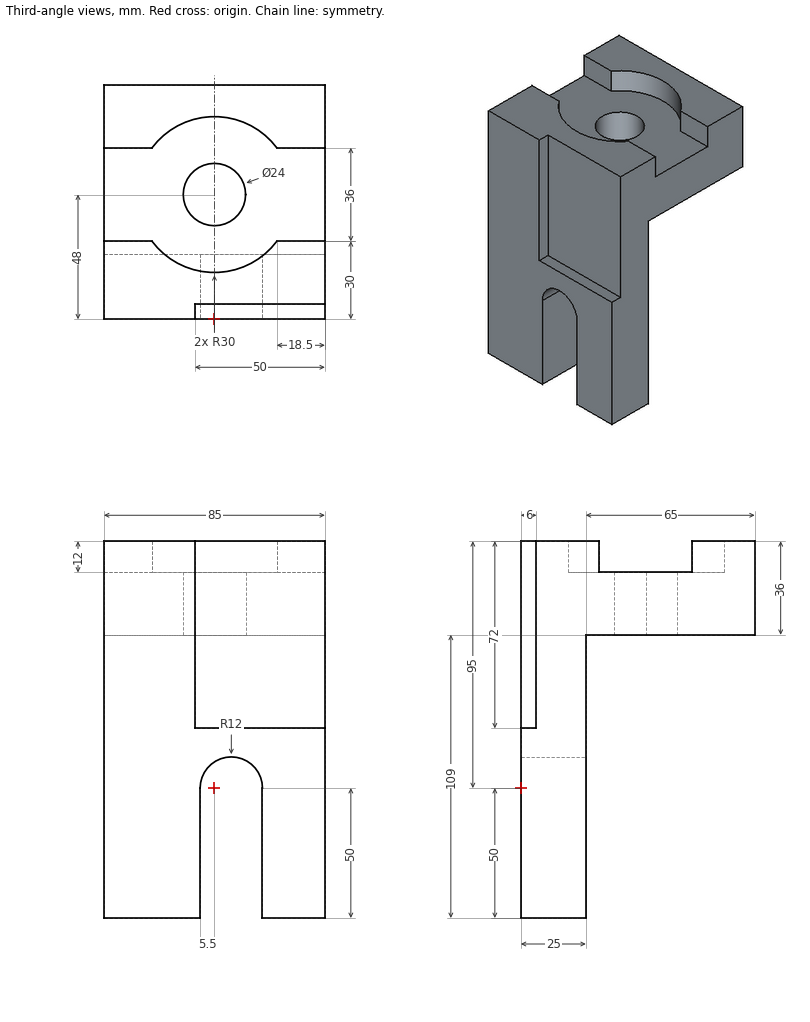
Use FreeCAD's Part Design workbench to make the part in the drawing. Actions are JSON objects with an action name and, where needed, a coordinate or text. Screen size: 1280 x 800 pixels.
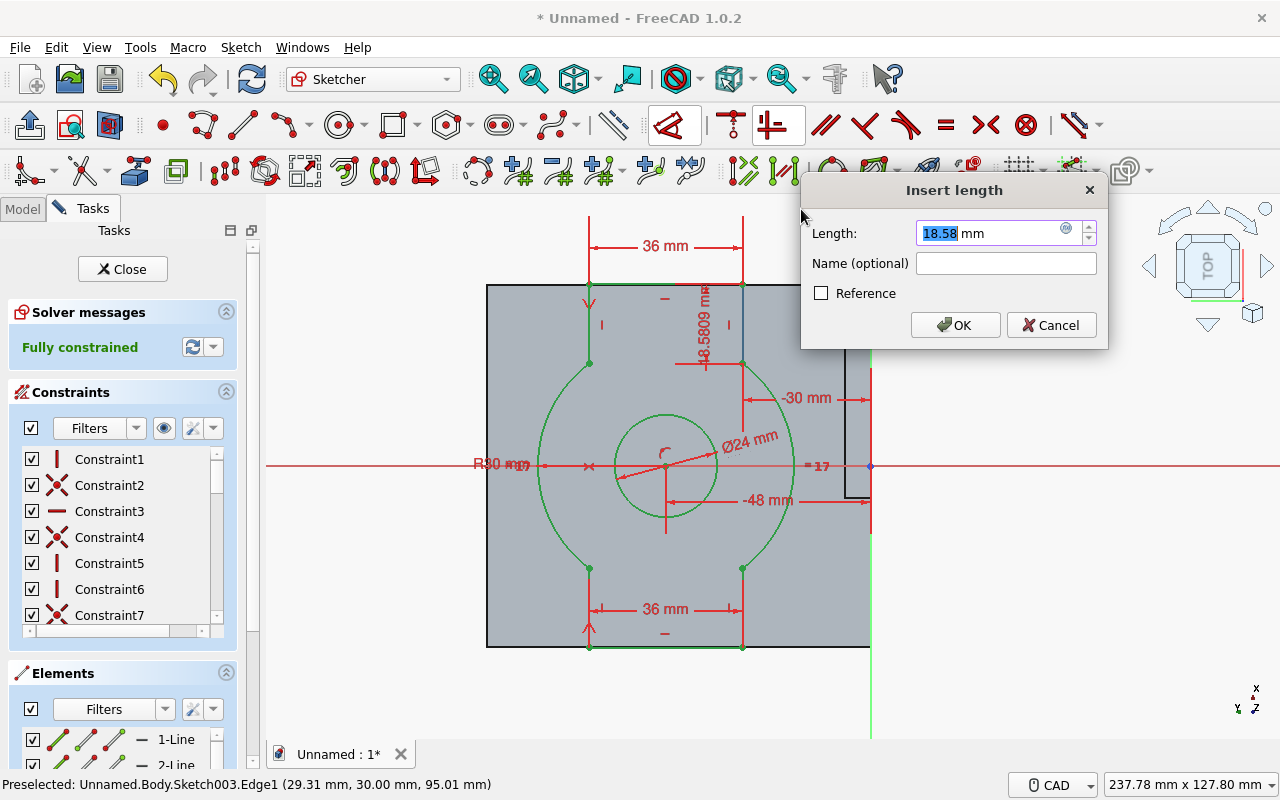
{"action": "type", "text": "18.5"}
{"action": "key", "text": "Return"}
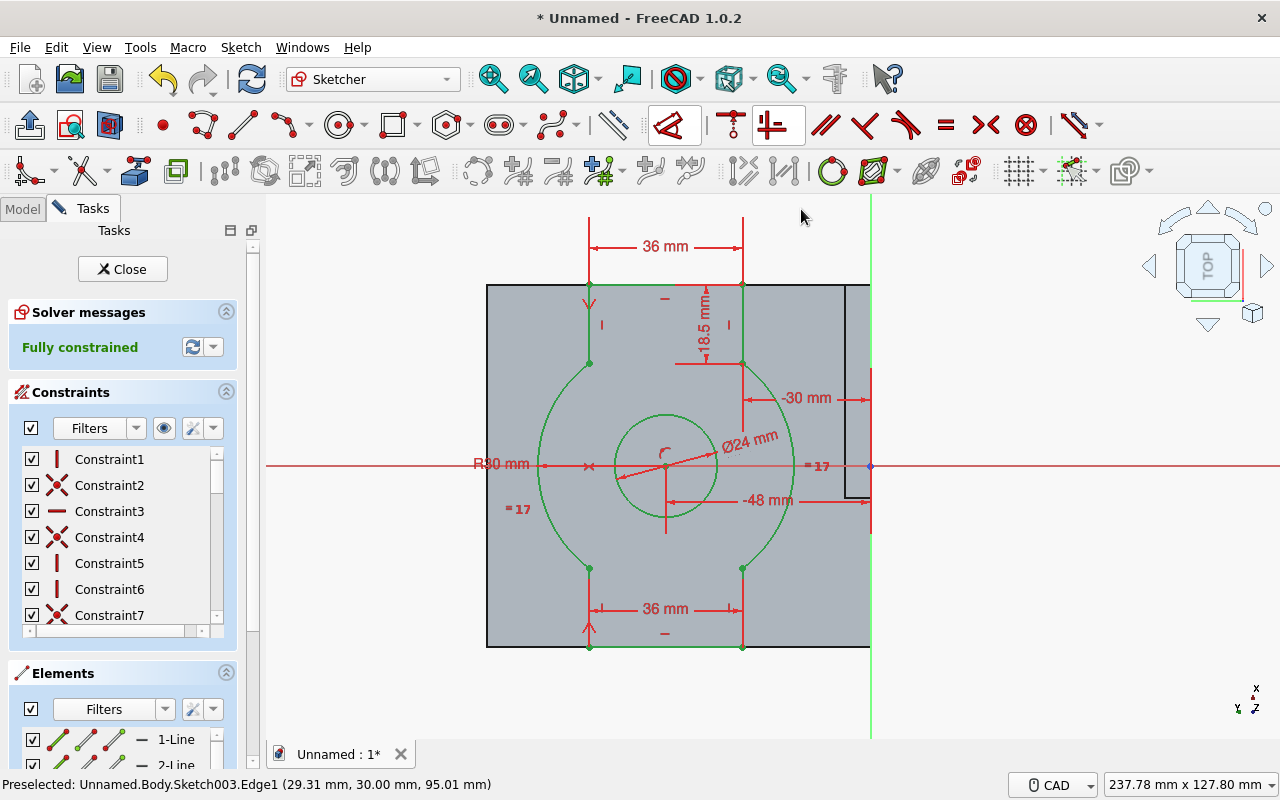
{"action": "left_click", "coordinate": [123, 269]}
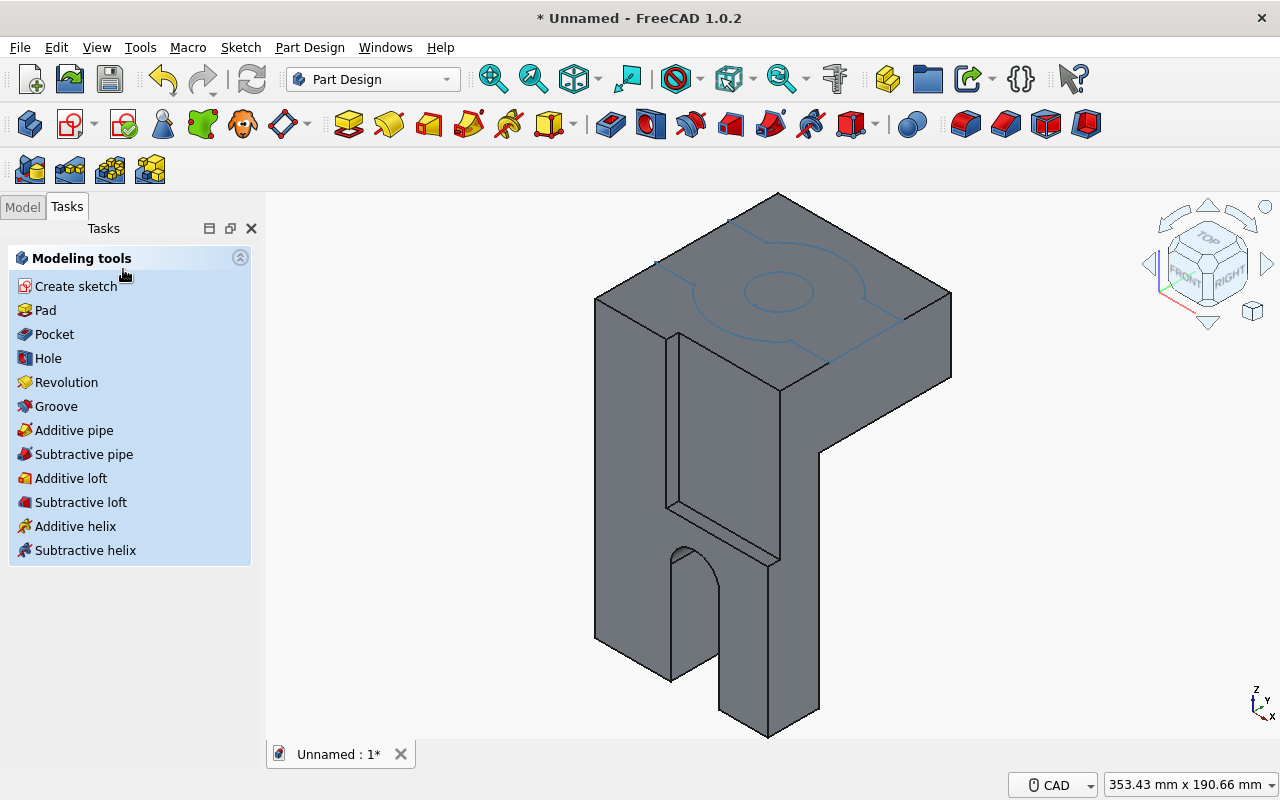
{"action": "left_click", "coordinate": [612, 124]}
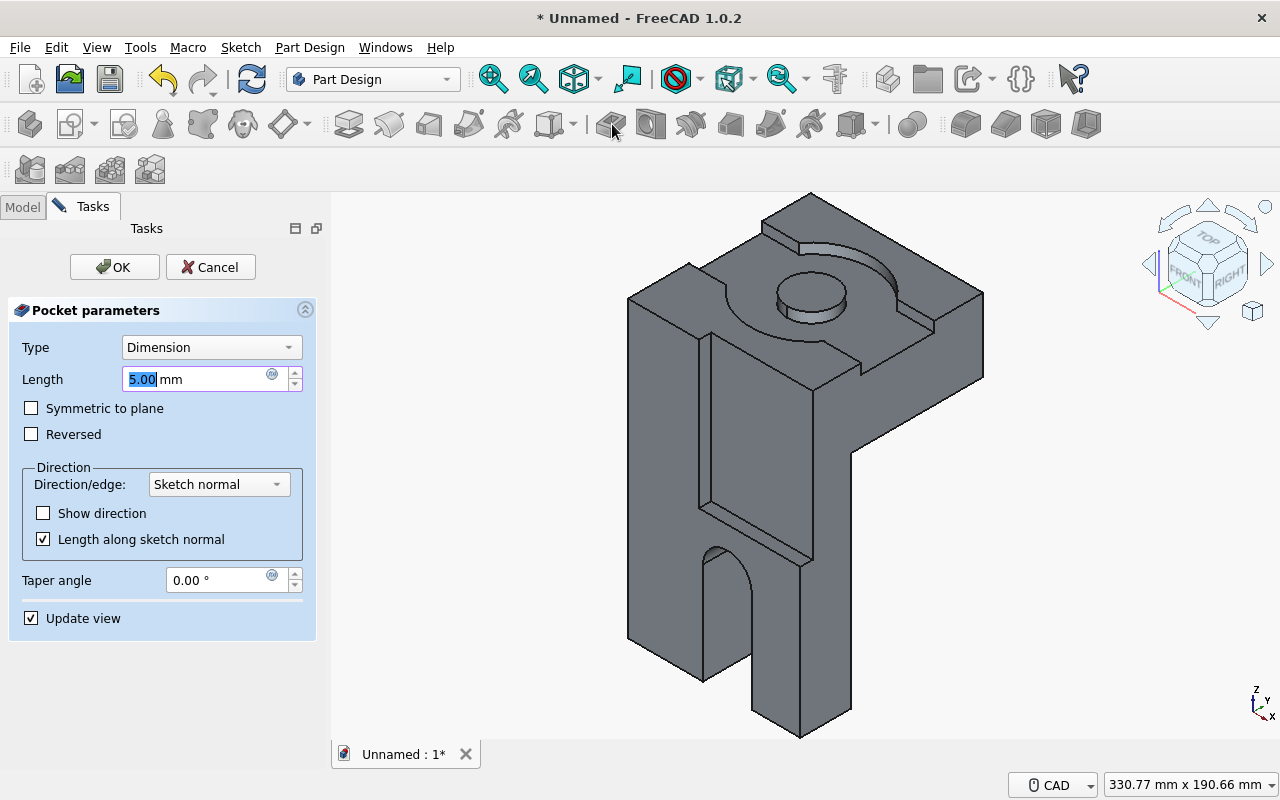
{"action": "type", "text": "12"}
{"action": "key", "text": "Tab"}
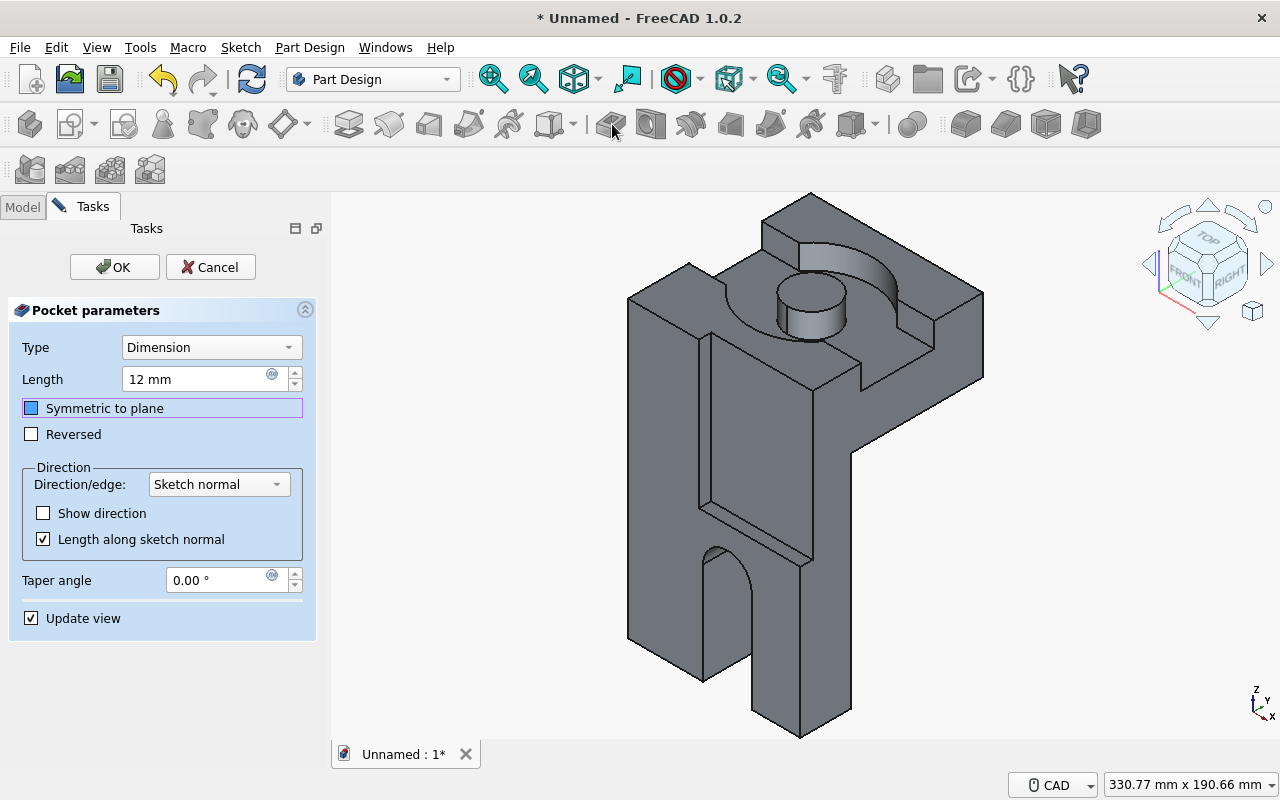
{"action": "left_click", "coordinate": [115, 267]}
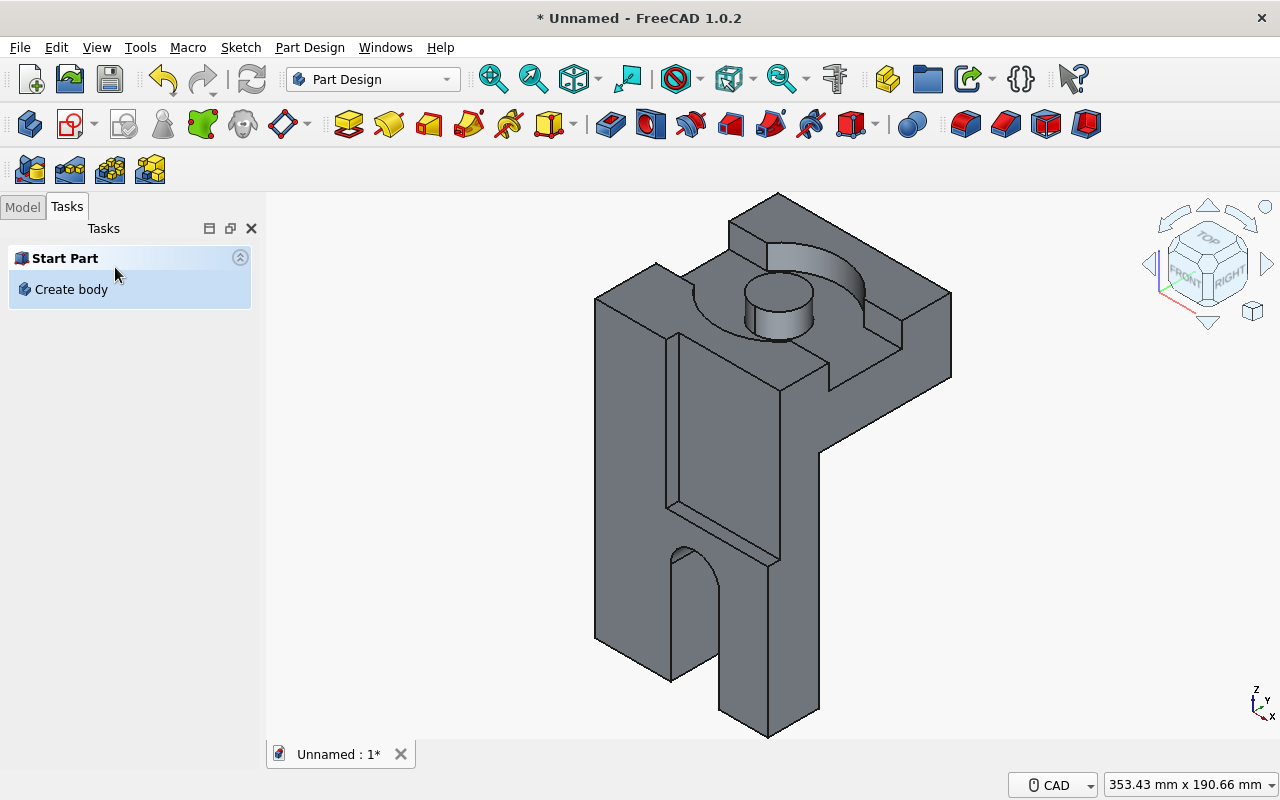
{"action": "left_click", "coordinate": [663, 301]}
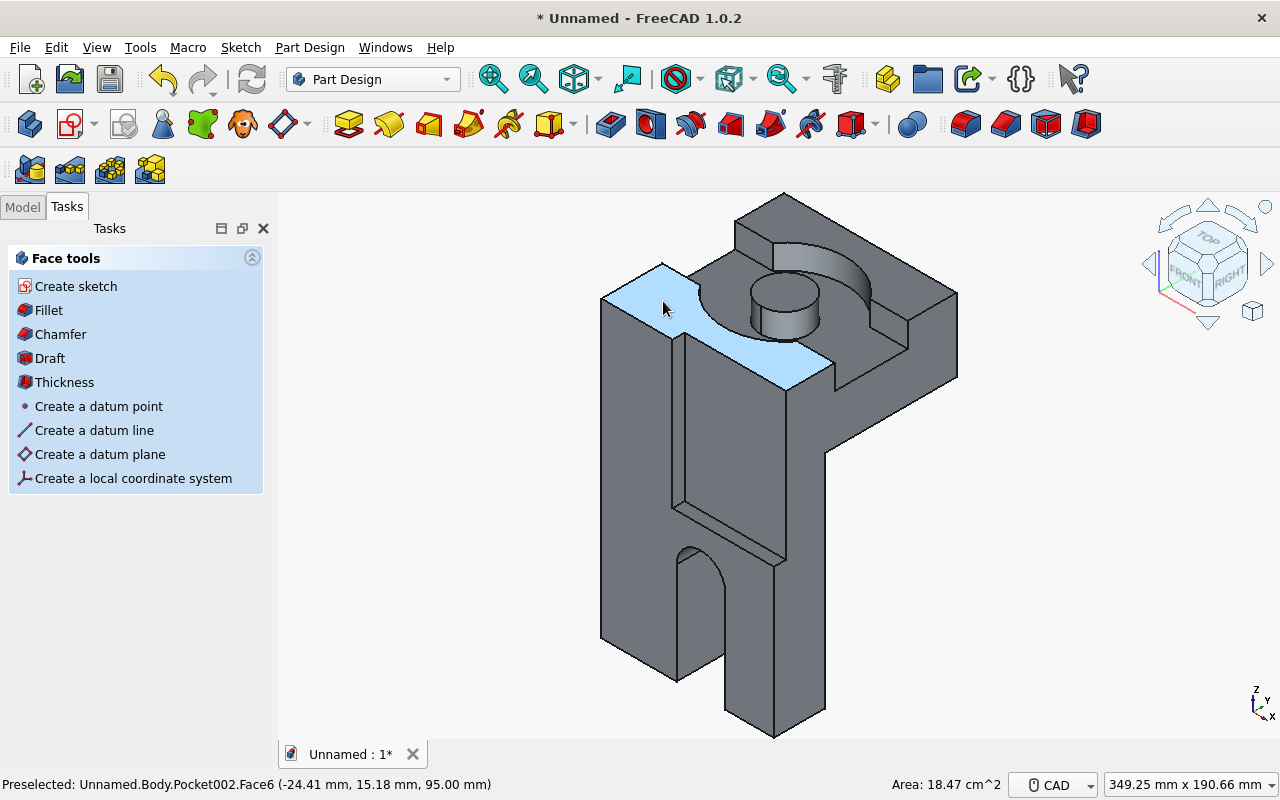
{"action": "left_click", "coordinate": [70, 124]}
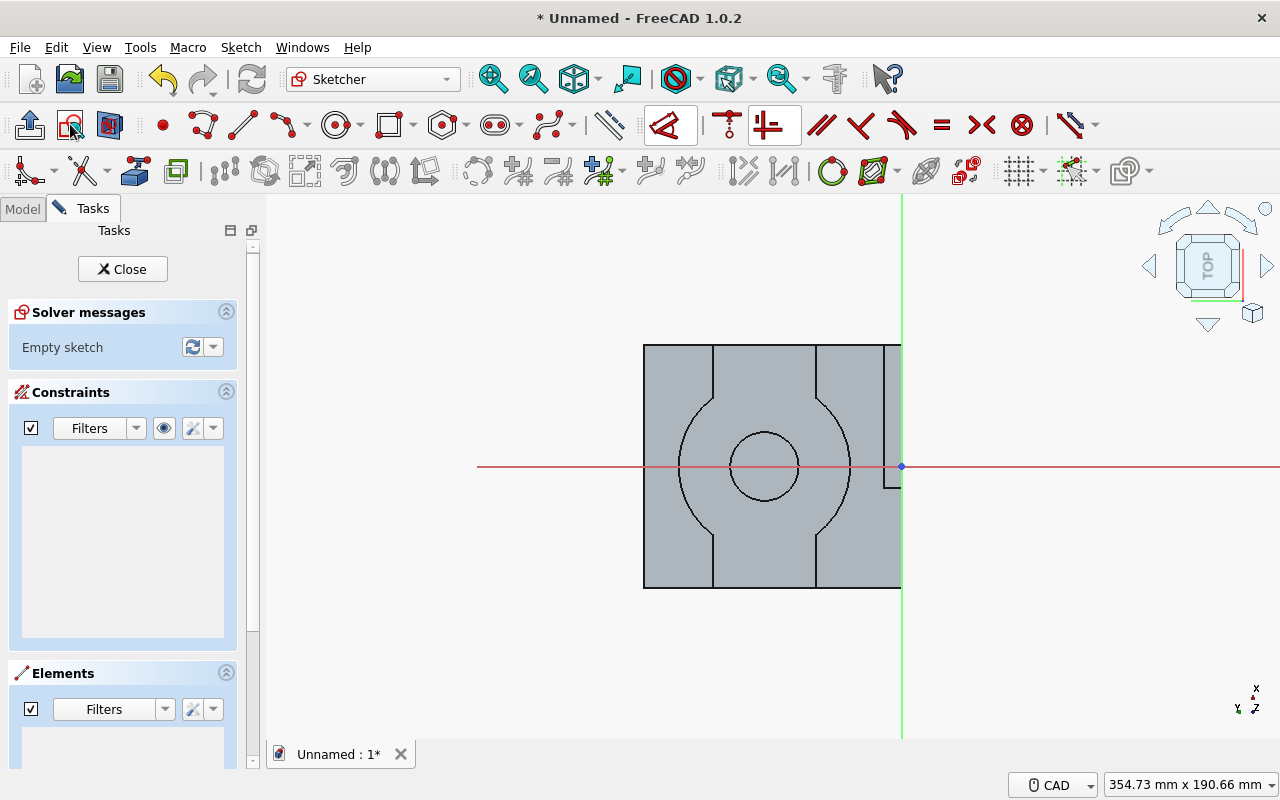
{"action": "scroll", "coordinate": [780, 467], "scroll_direction": "up", "scroll_amount": 8}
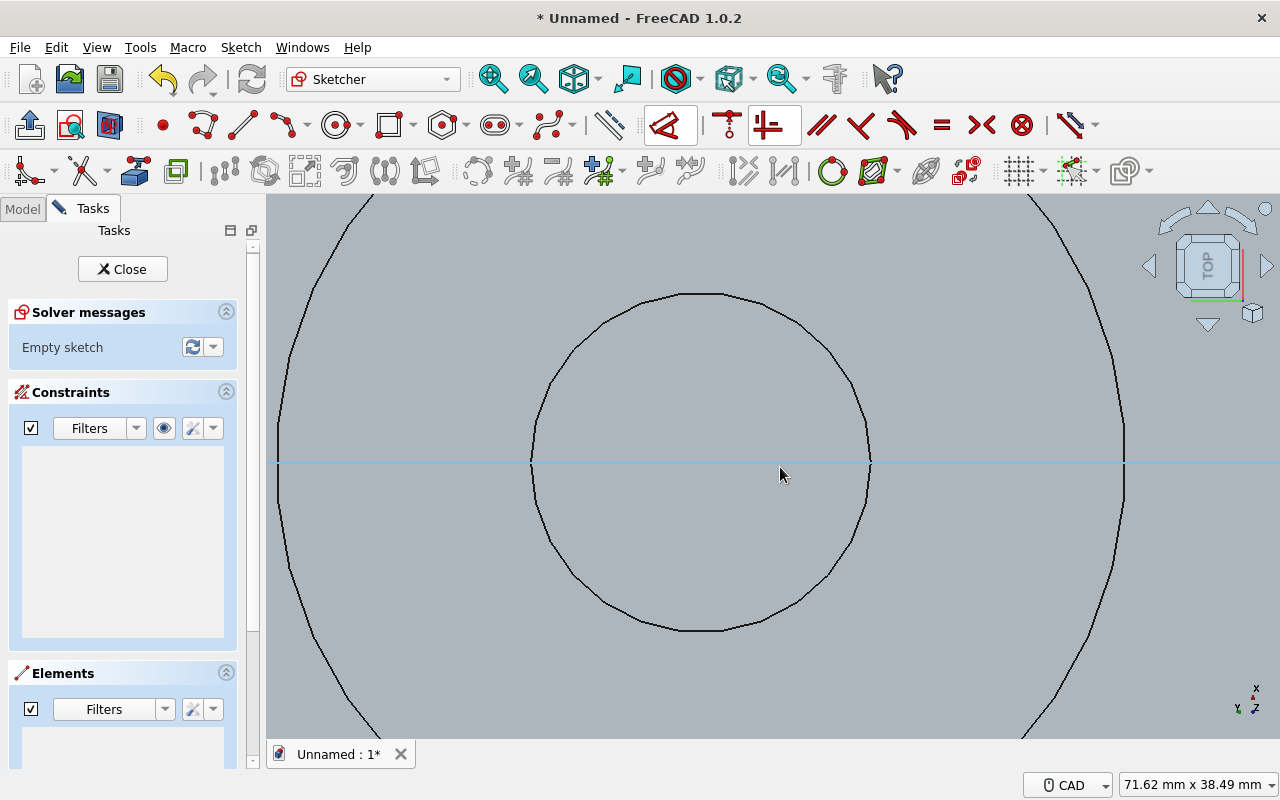
{"action": "left_click", "coordinate": [336, 126]}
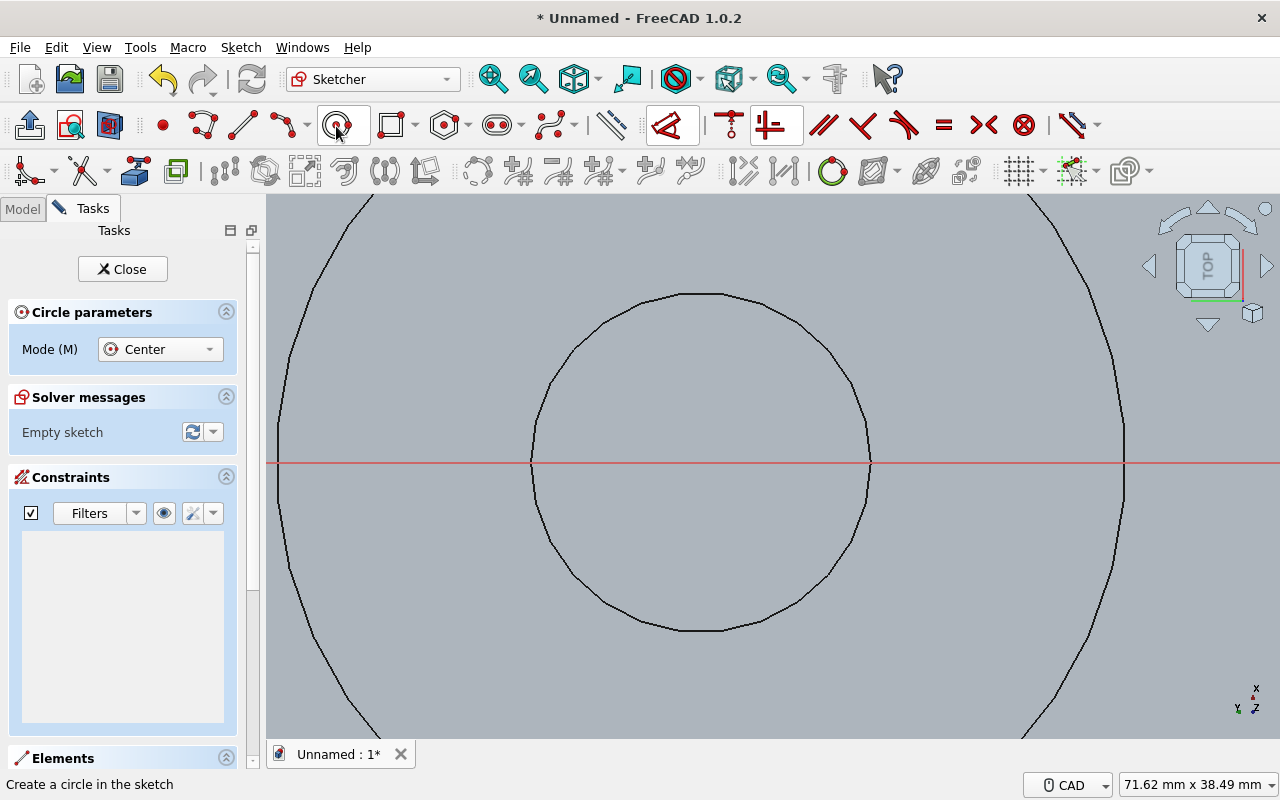
{"action": "left_click", "coordinate": [701, 463]}
{"action": "left_click", "coordinate": [821, 342]}
{"action": "key", "text": "Escape"}